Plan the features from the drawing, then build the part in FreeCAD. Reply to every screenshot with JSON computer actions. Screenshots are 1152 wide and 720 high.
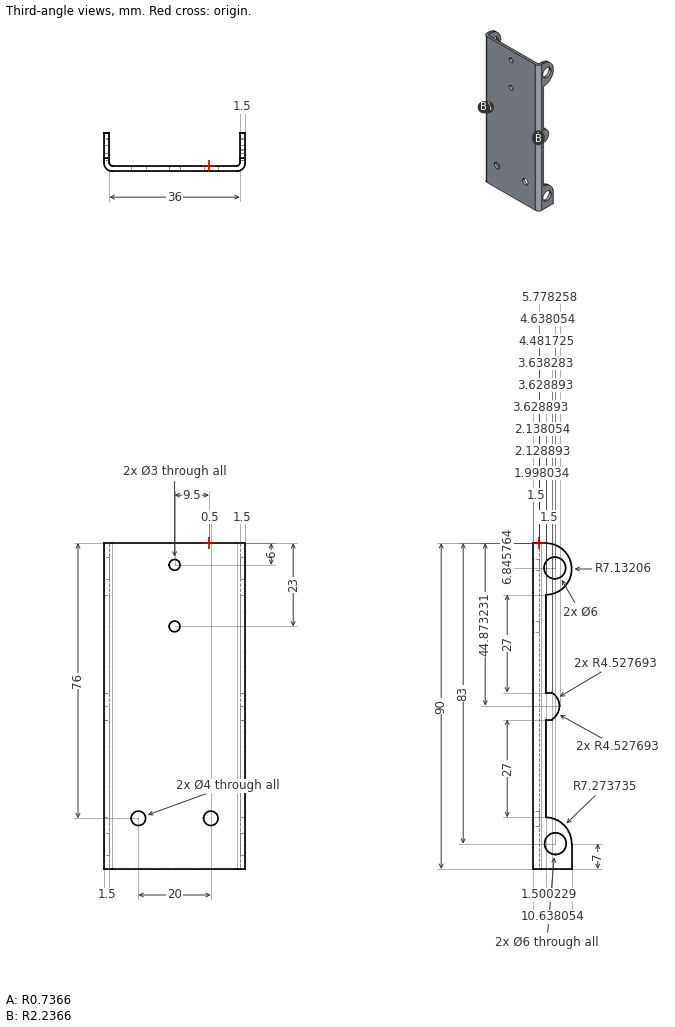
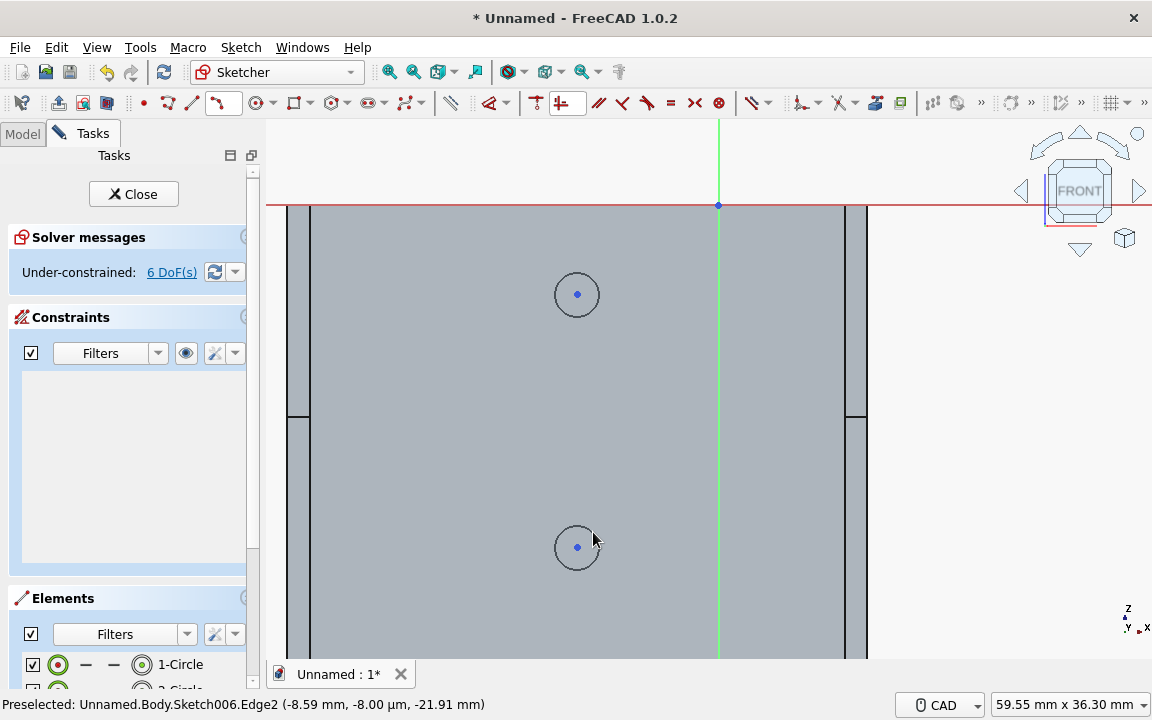
{"action": "left_click", "coordinate": [592, 279]}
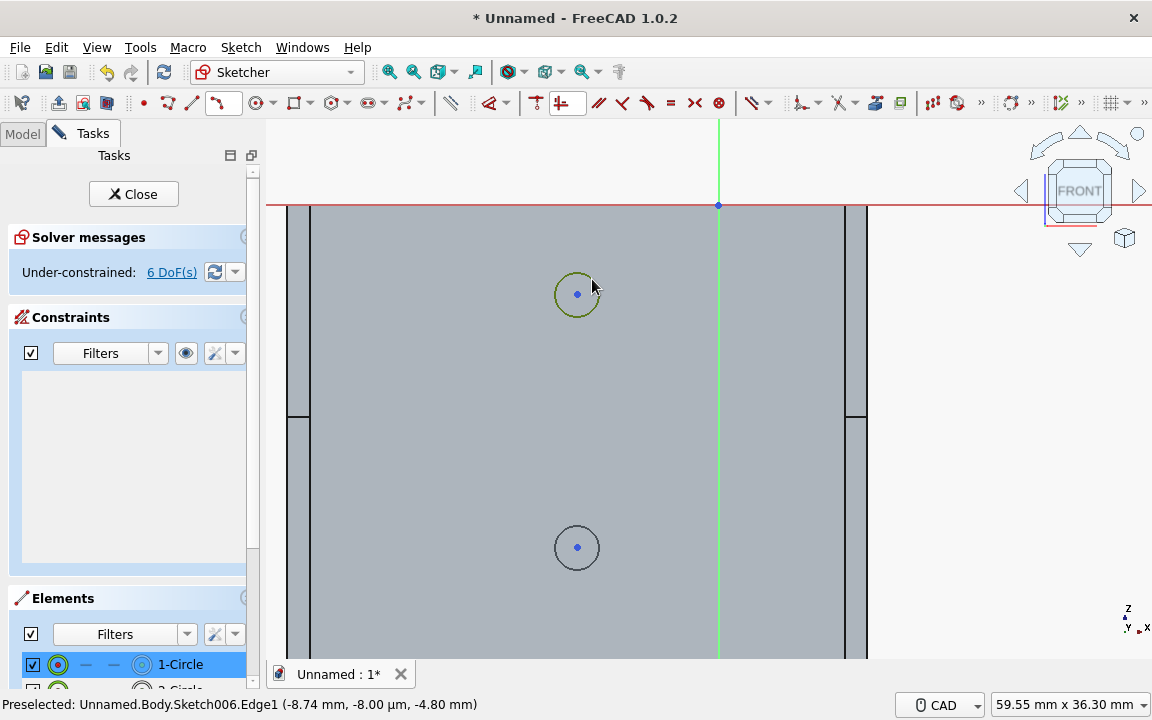
{"action": "left_click", "coordinate": [592, 532]}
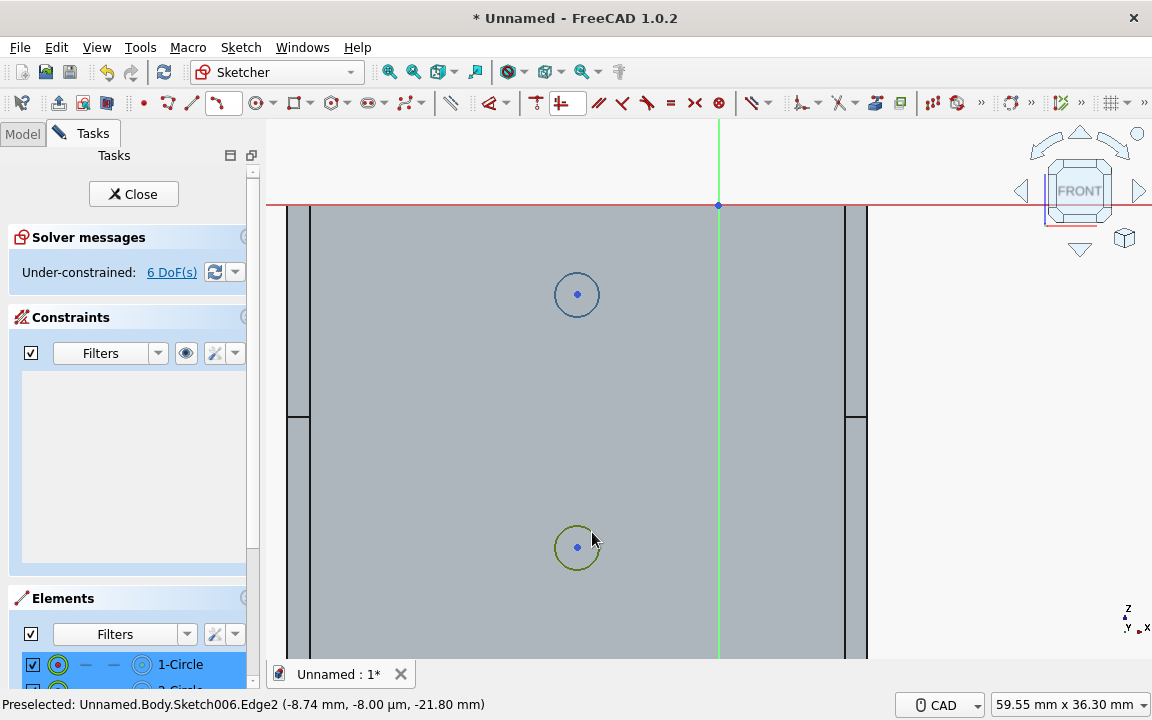
{"action": "key", "text": "e"}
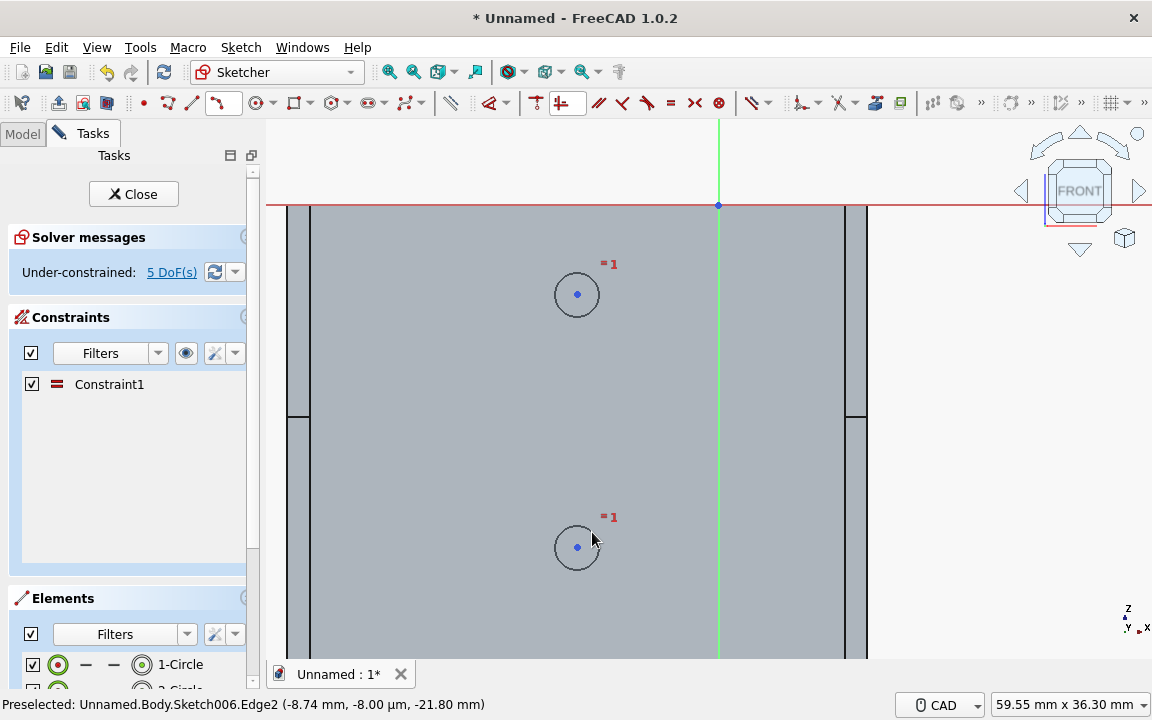
{"action": "left_click", "coordinate": [577, 295]}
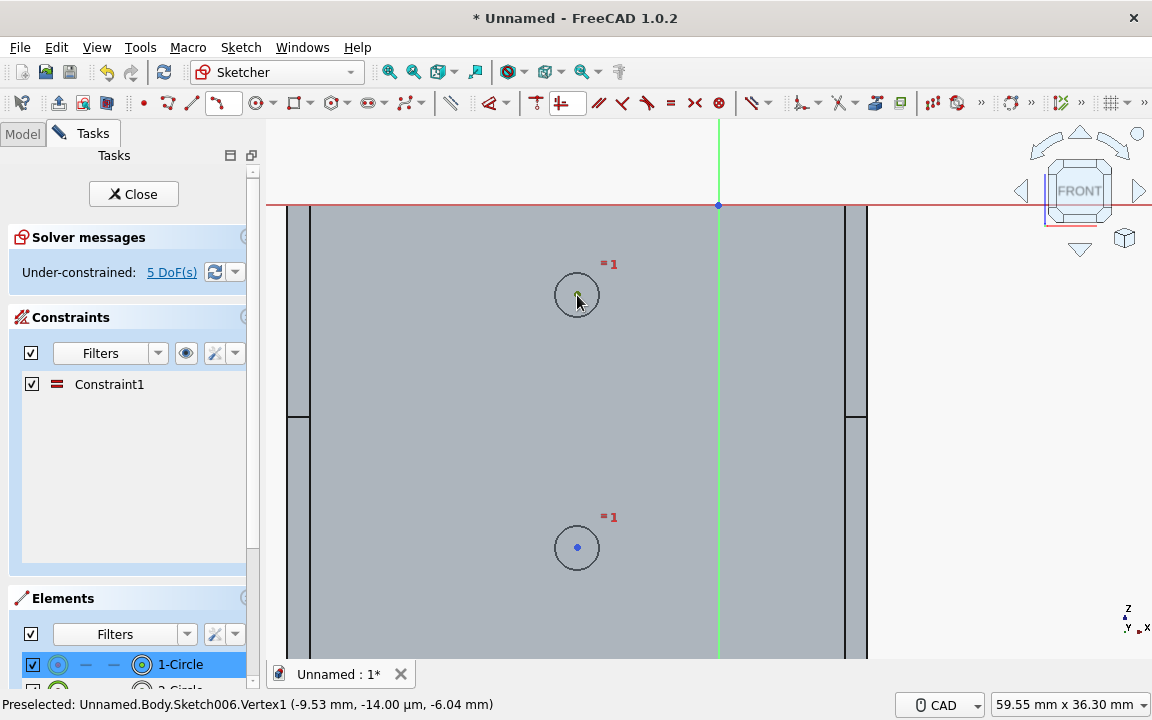
{"action": "left_click", "coordinate": [577, 548]}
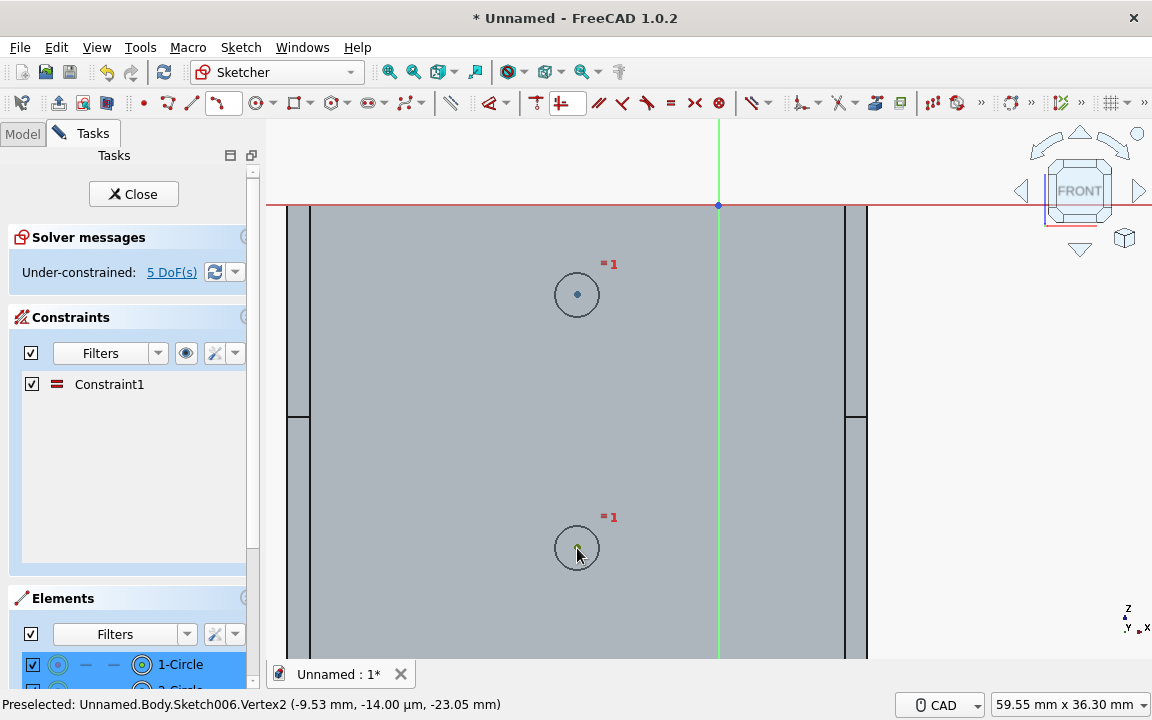
{"action": "key", "text": "v"}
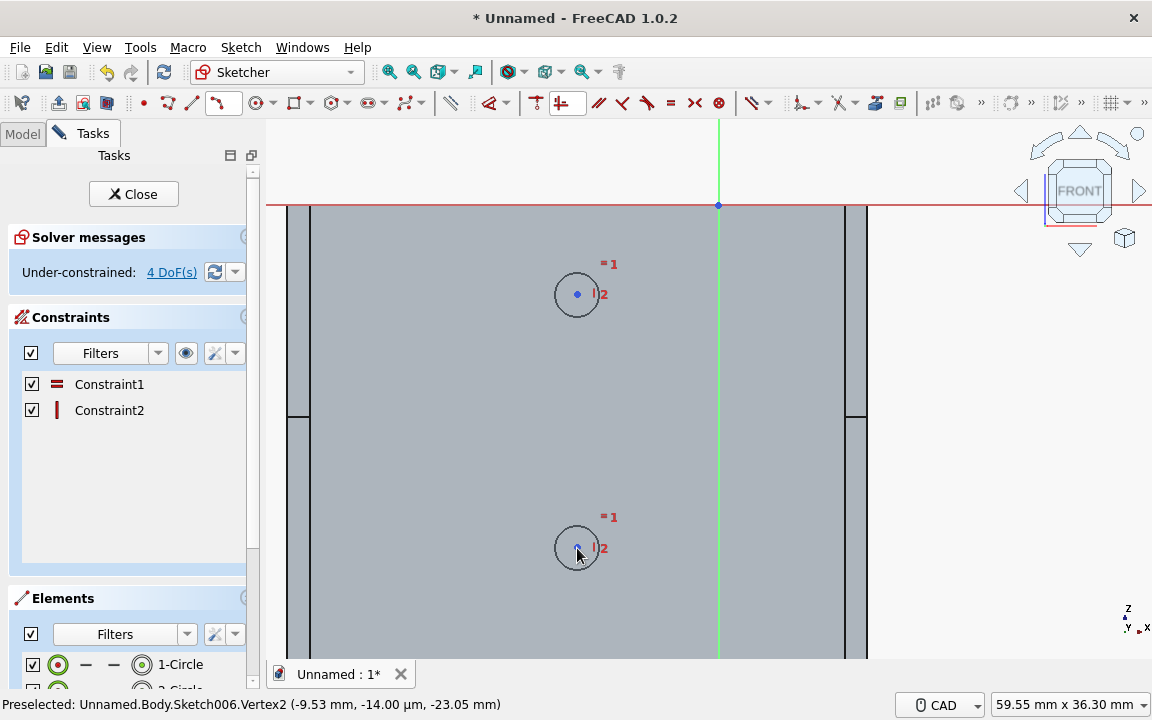
{"action": "key", "text": "d"}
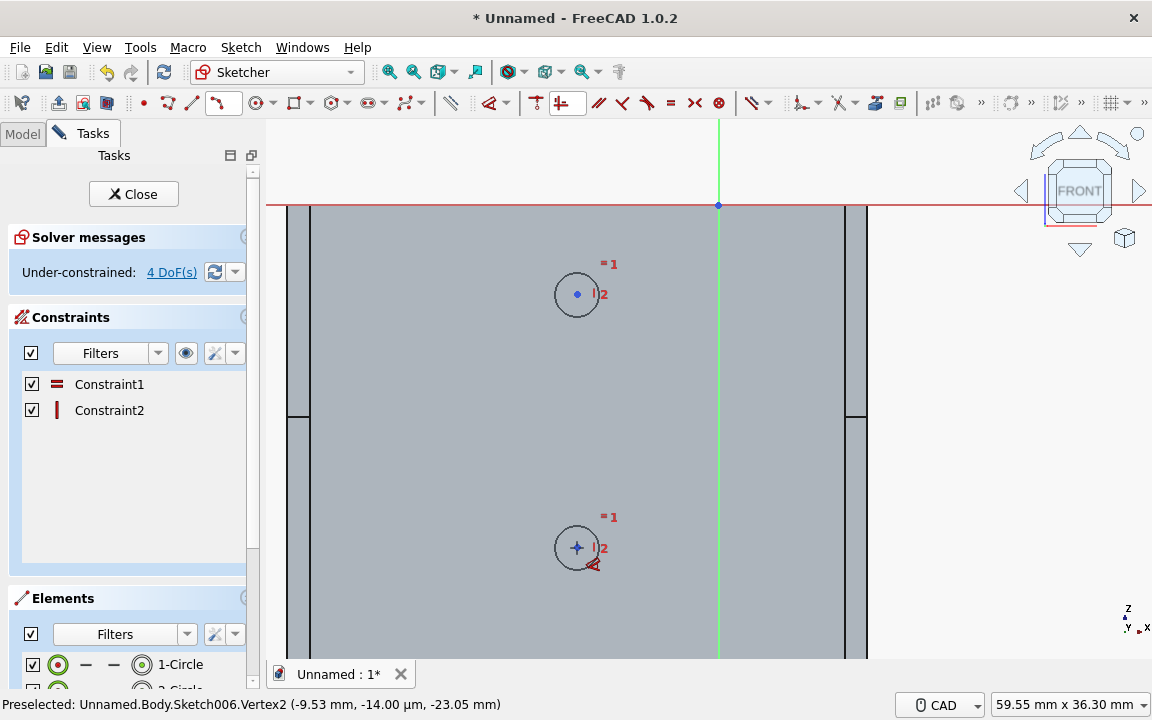
{"action": "left_click", "coordinate": [592, 279]}
{"action": "left_click", "coordinate": [614, 256]}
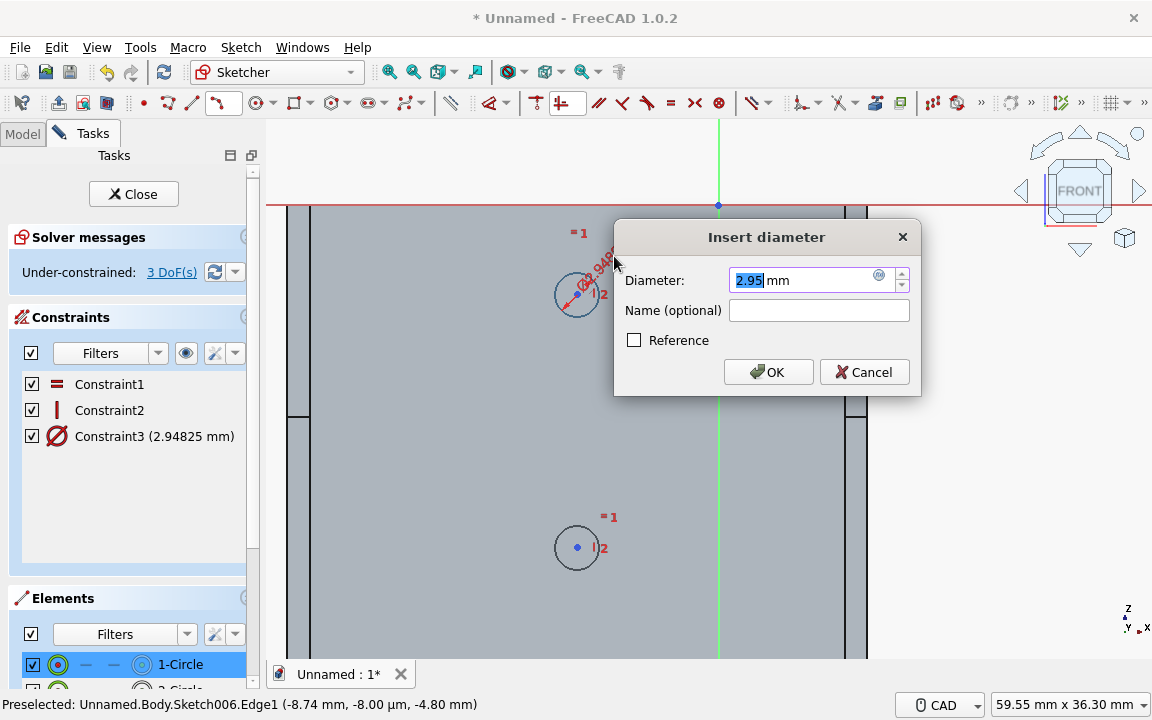
{"action": "type", "text": "3"}
{"action": "key", "text": "Return"}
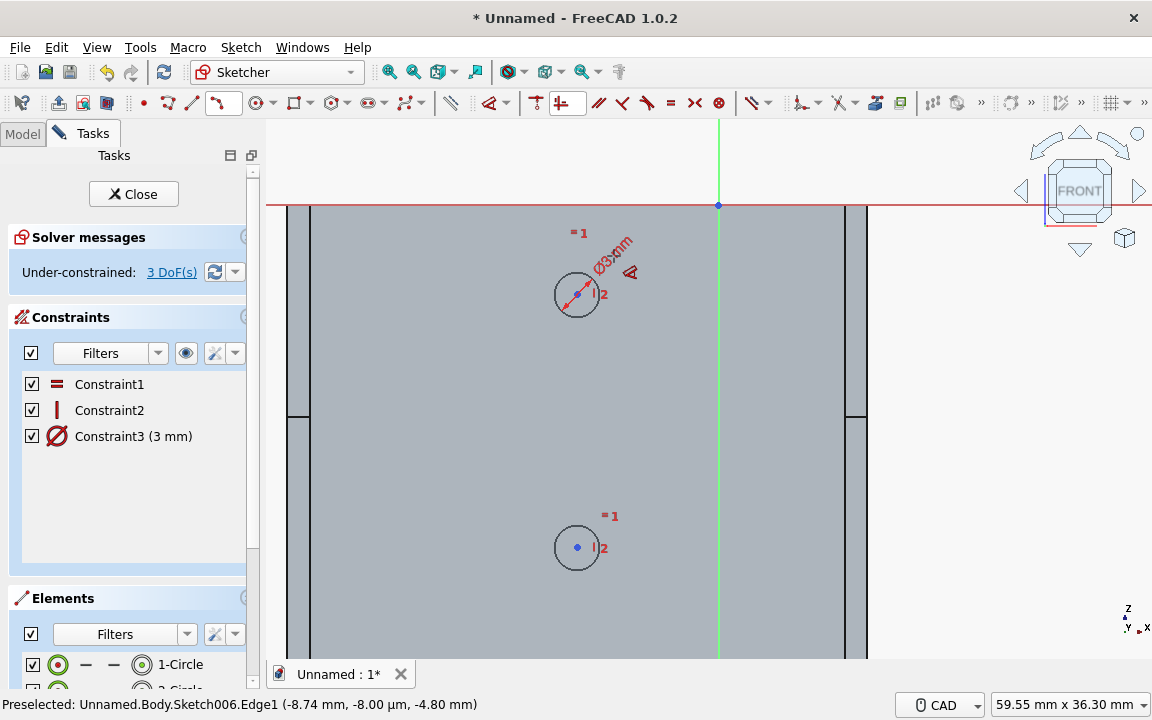
{"action": "left_click", "coordinate": [577, 295]}
{"action": "left_click", "coordinate": [753, 250]}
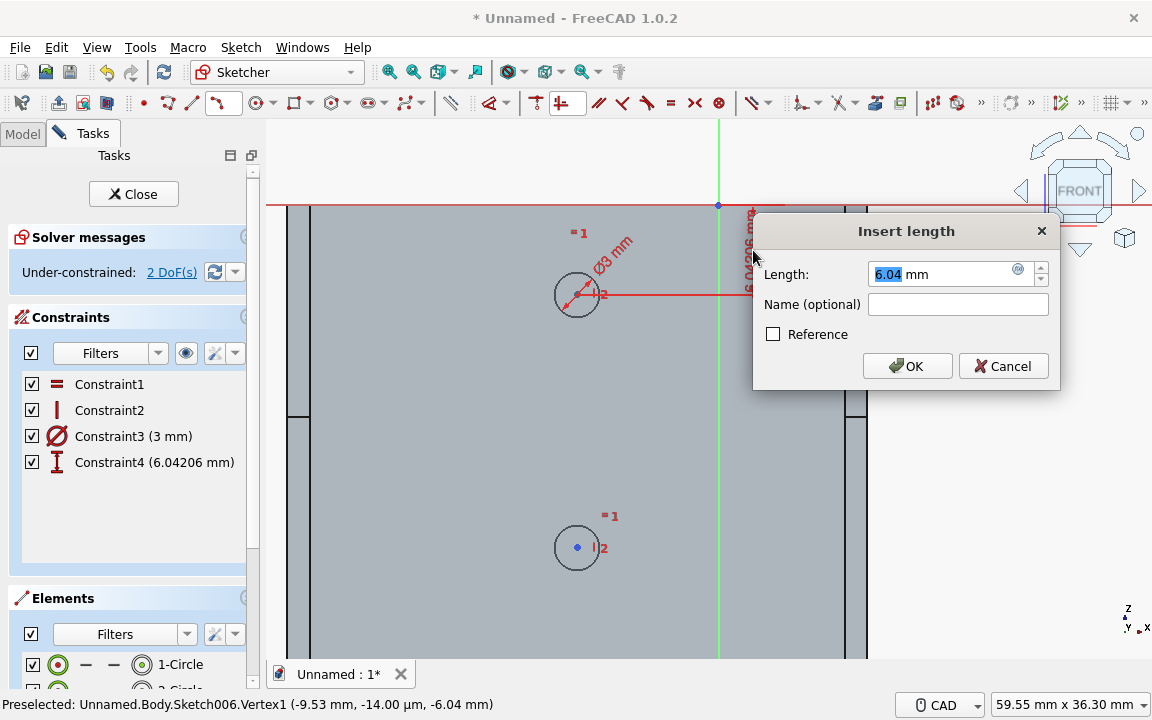
{"action": "type", "text": "6"}
{"action": "key", "text": "Return"}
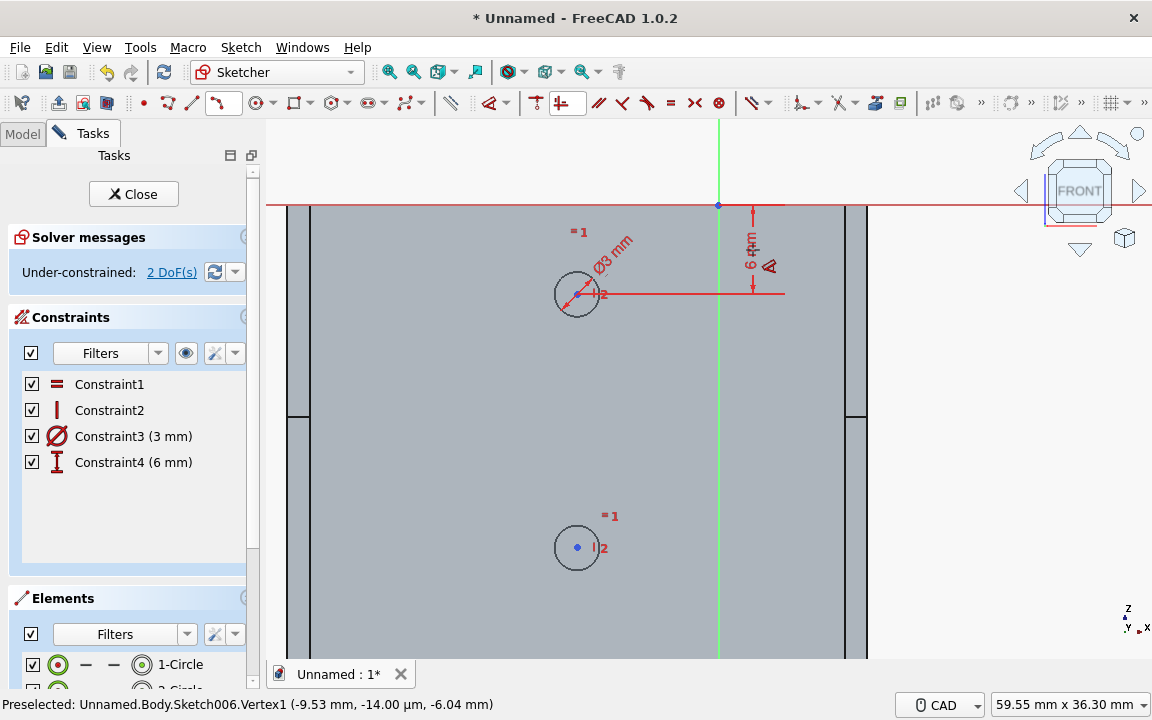
{"action": "left_click", "coordinate": [577, 548]}
{"action": "left_click", "coordinate": [753, 377]}